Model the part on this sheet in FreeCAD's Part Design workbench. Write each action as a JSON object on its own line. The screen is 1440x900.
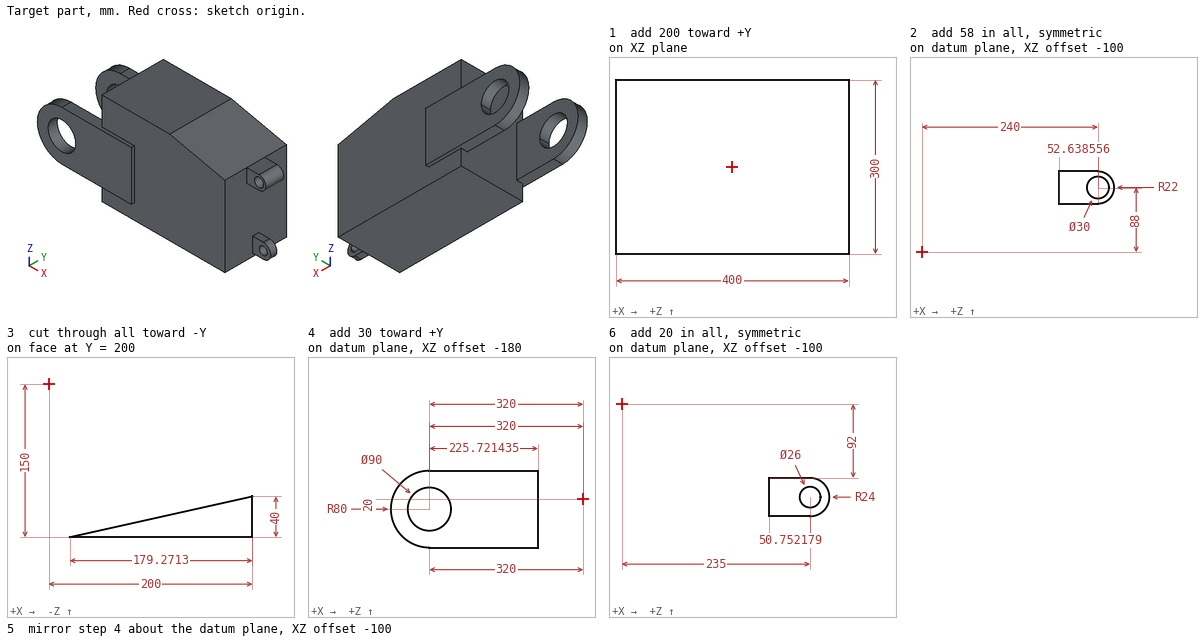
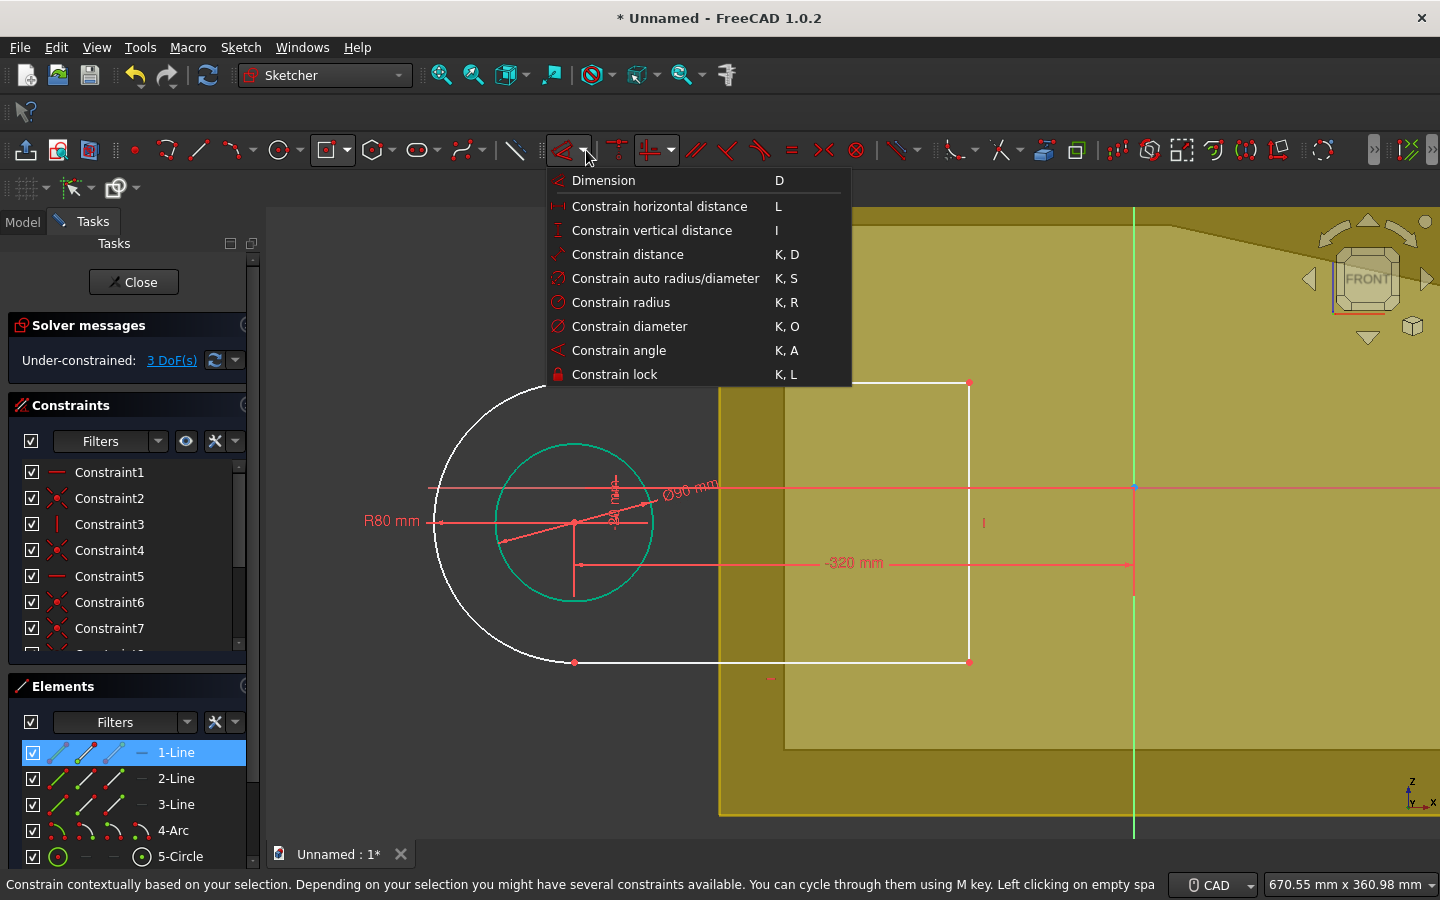
{"action": "left_click", "coordinate": [699, 206]}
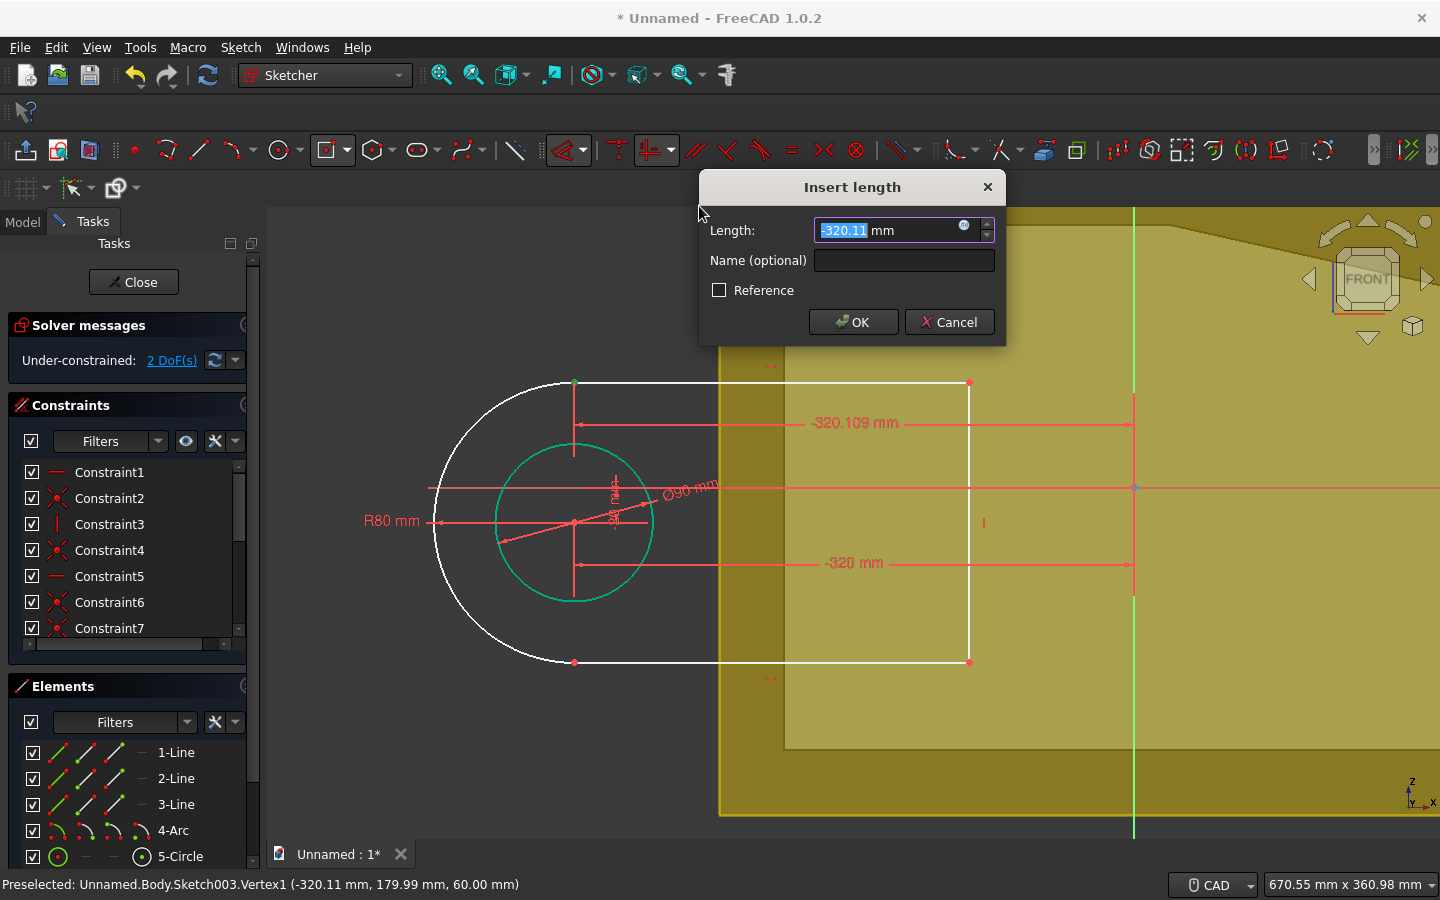
{"action": "type", "text": "-320"}
{"action": "key", "text": "Return"}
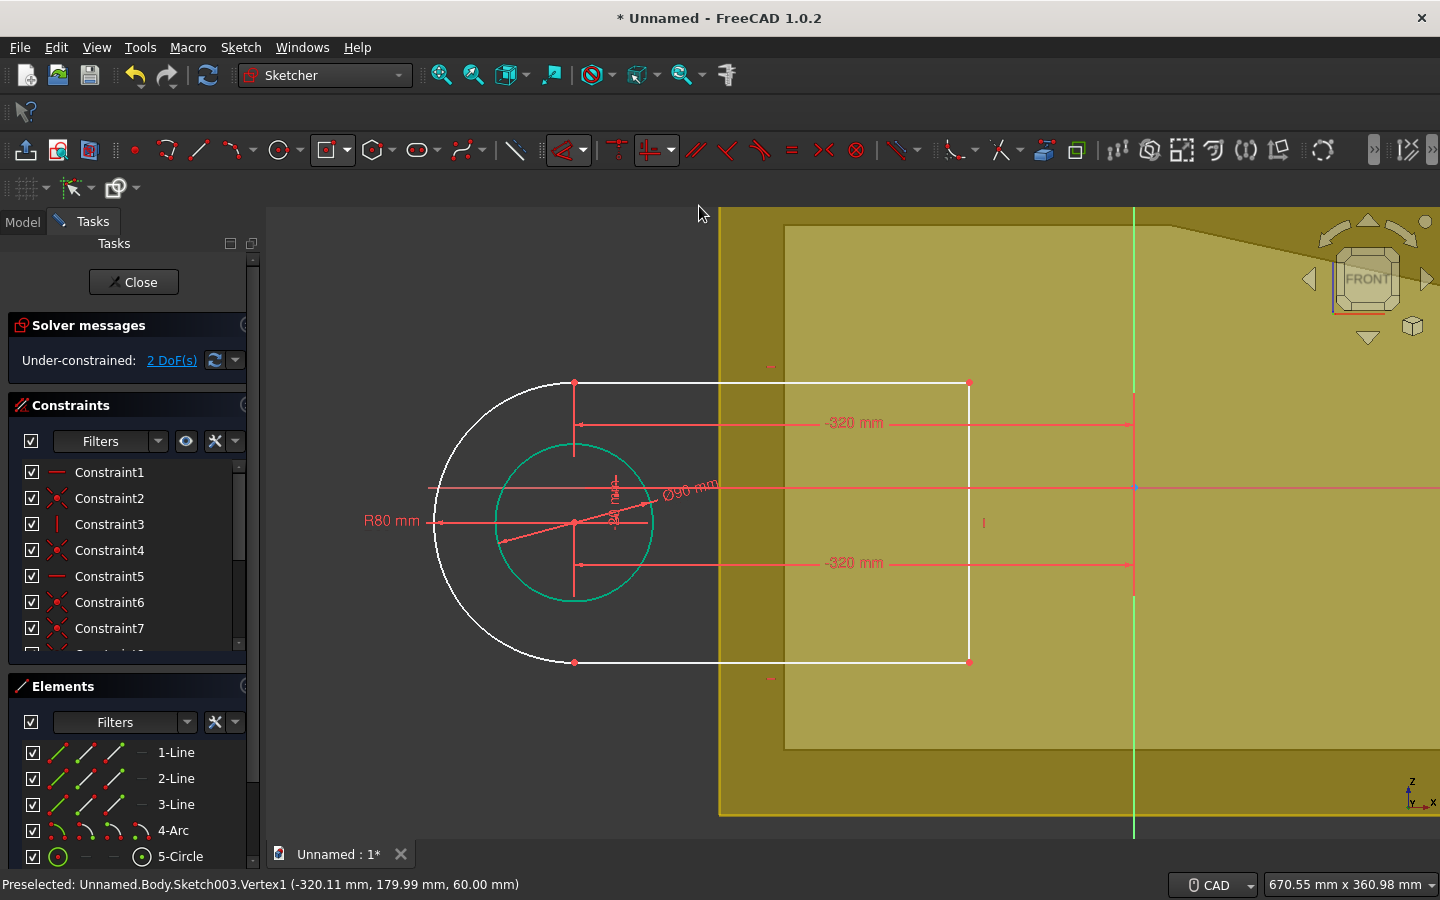
{"action": "left_click", "coordinate": [574, 663]}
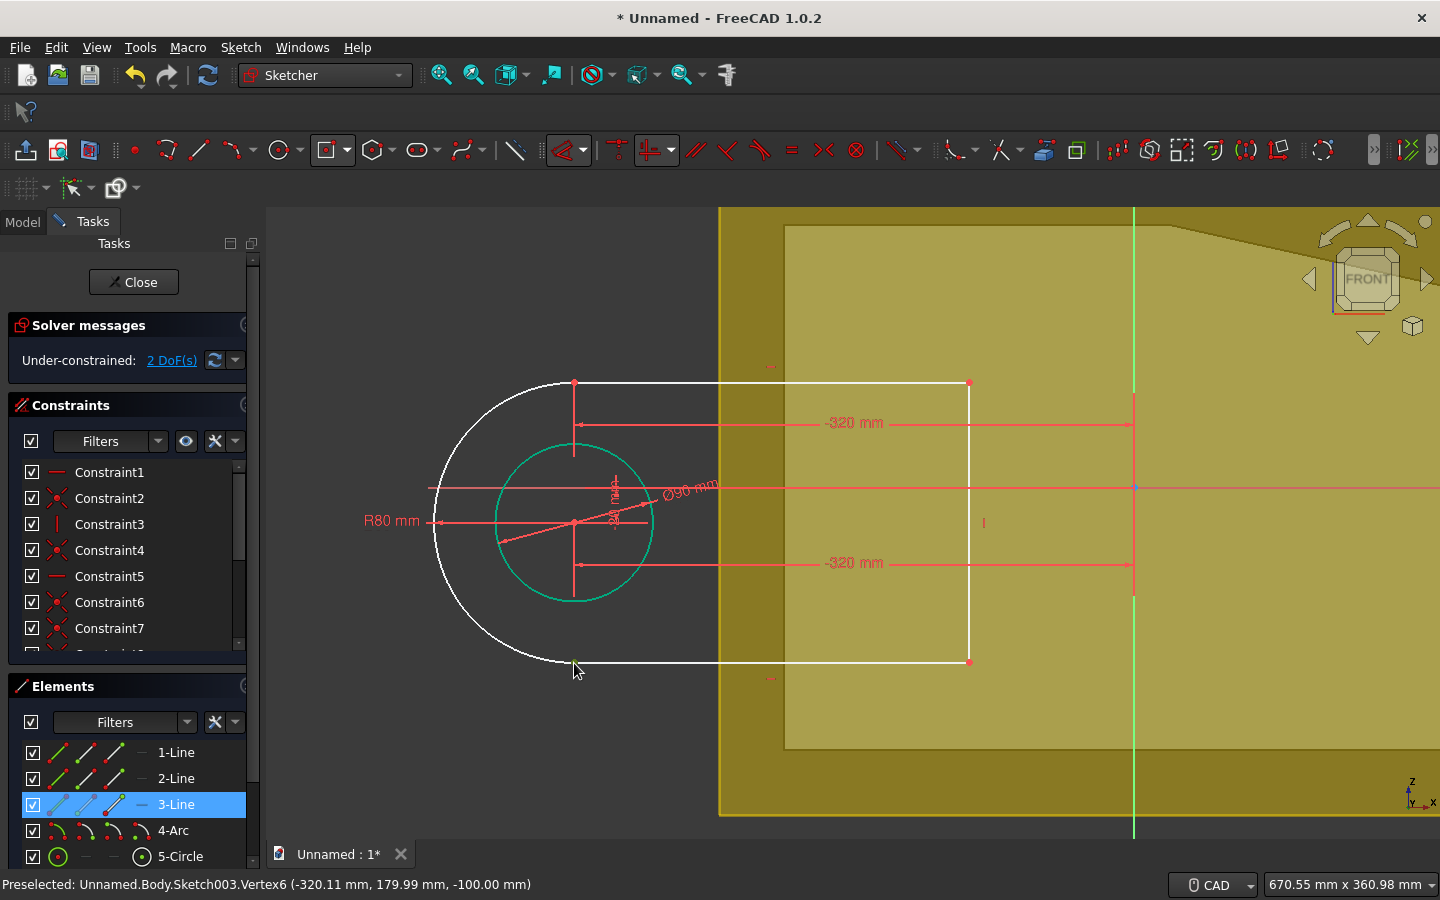
{"action": "left_click", "coordinate": [586, 150]}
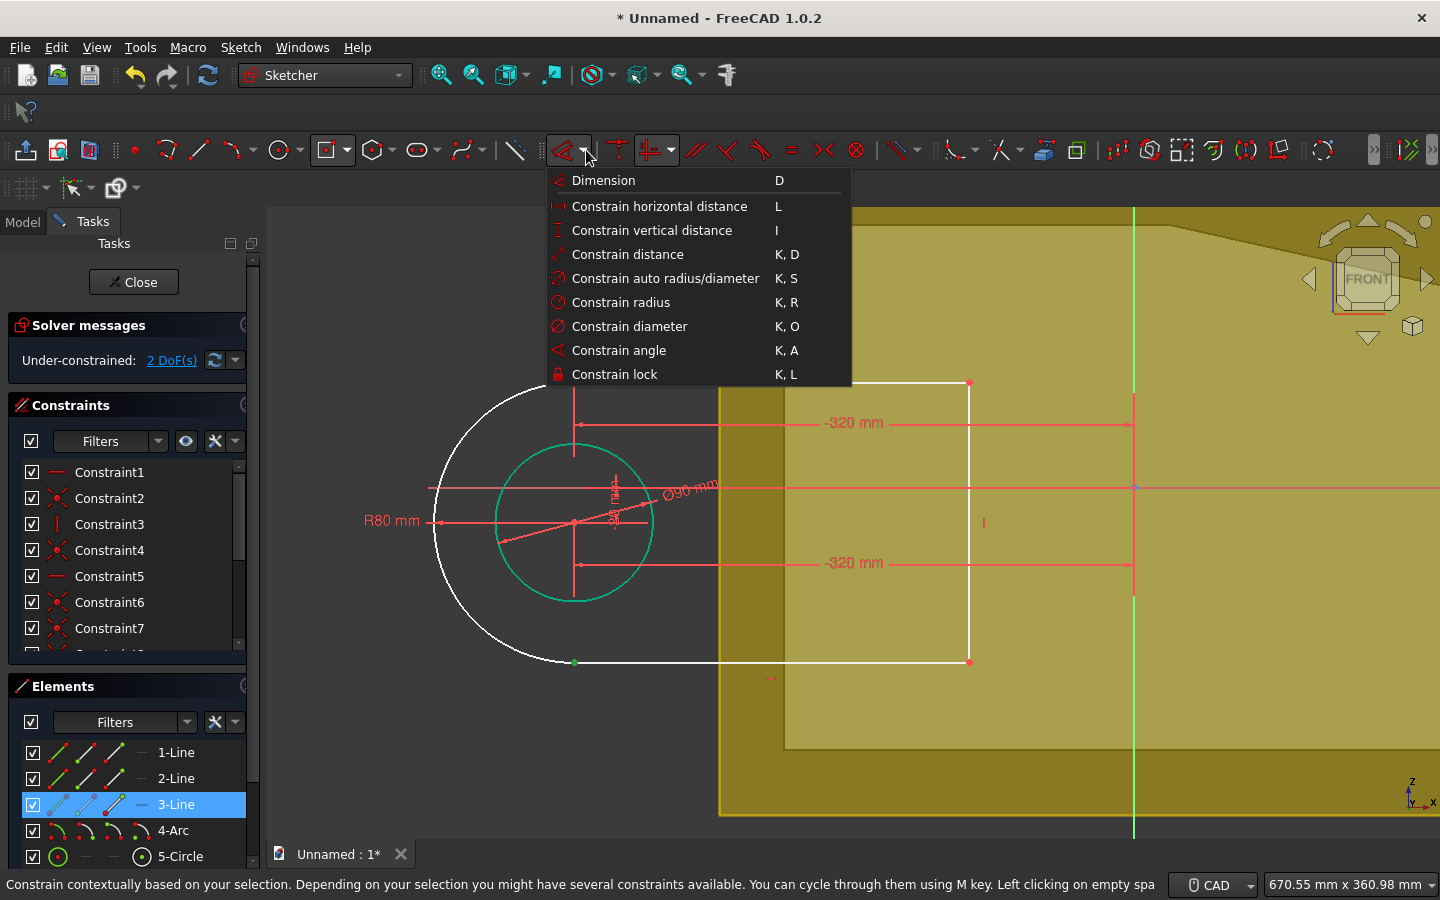
{"action": "left_click", "coordinate": [699, 206]}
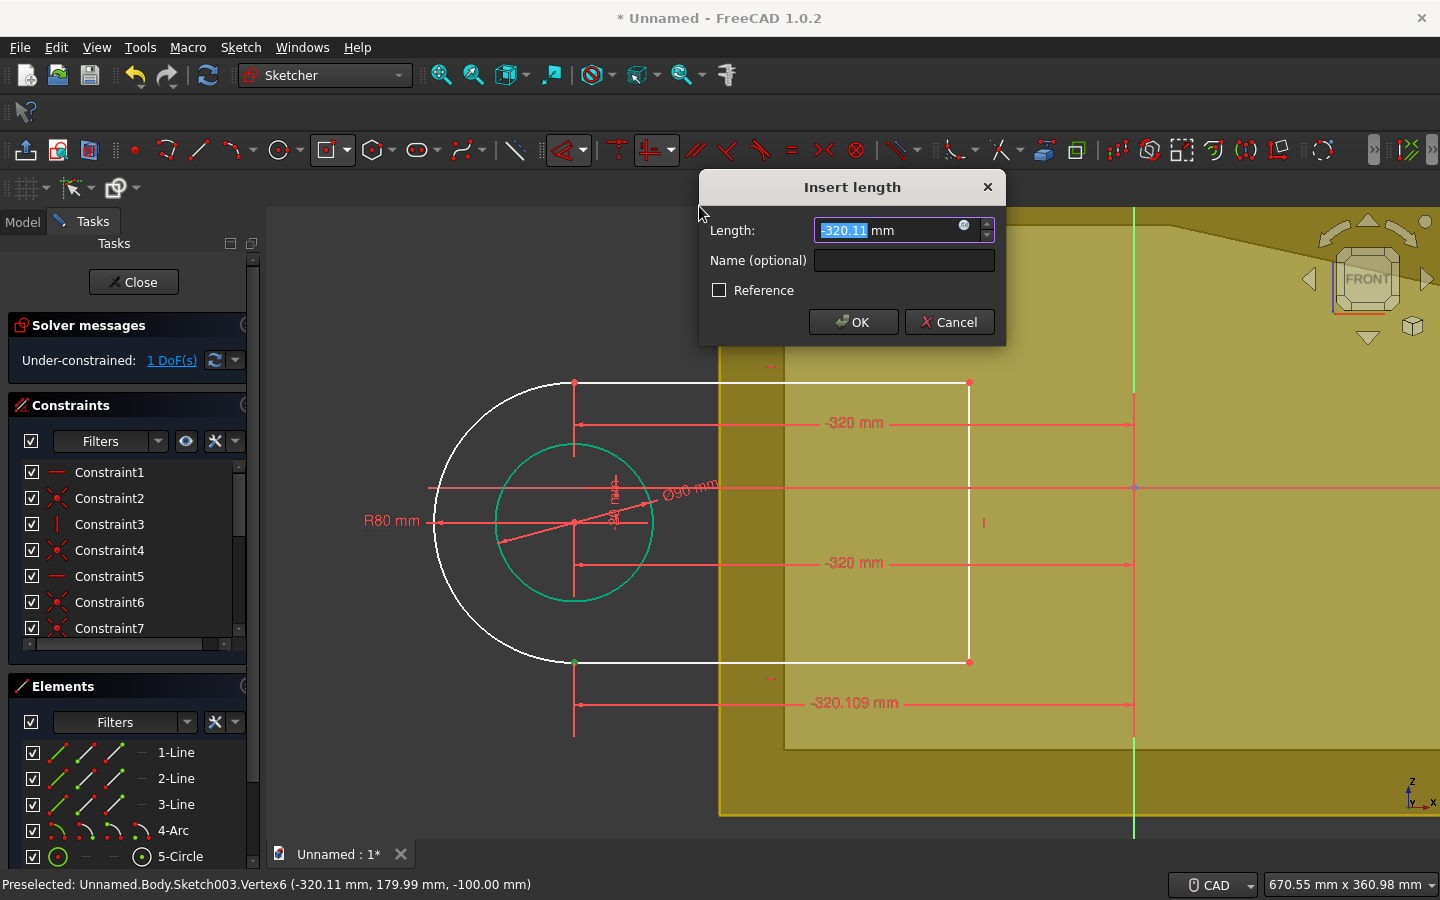
{"action": "type", "text": "-320"}
{"action": "key", "text": "Return"}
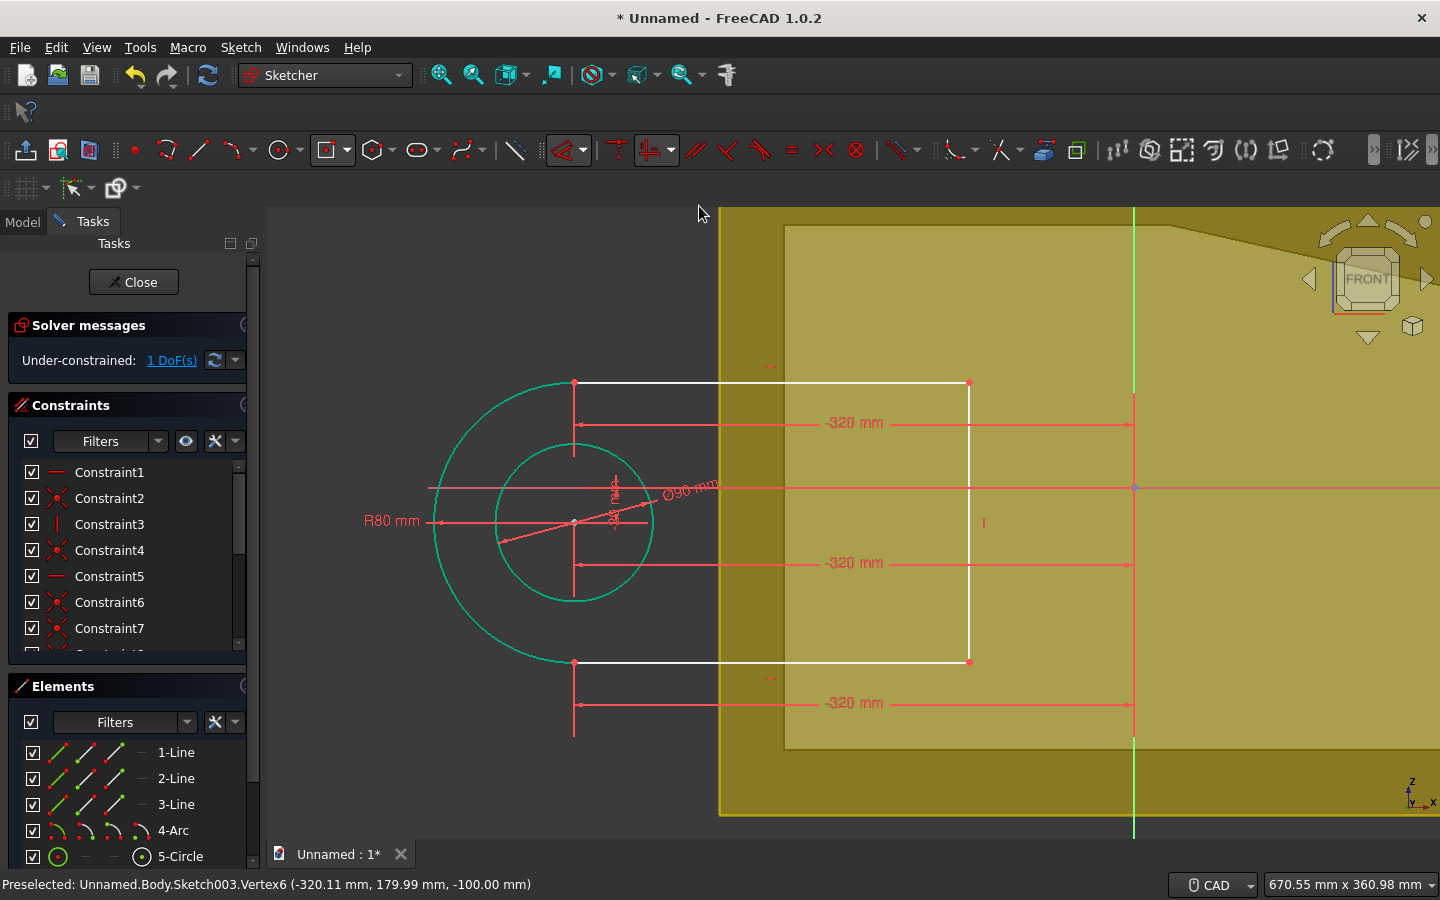
{"action": "left_click", "coordinate": [693, 383]}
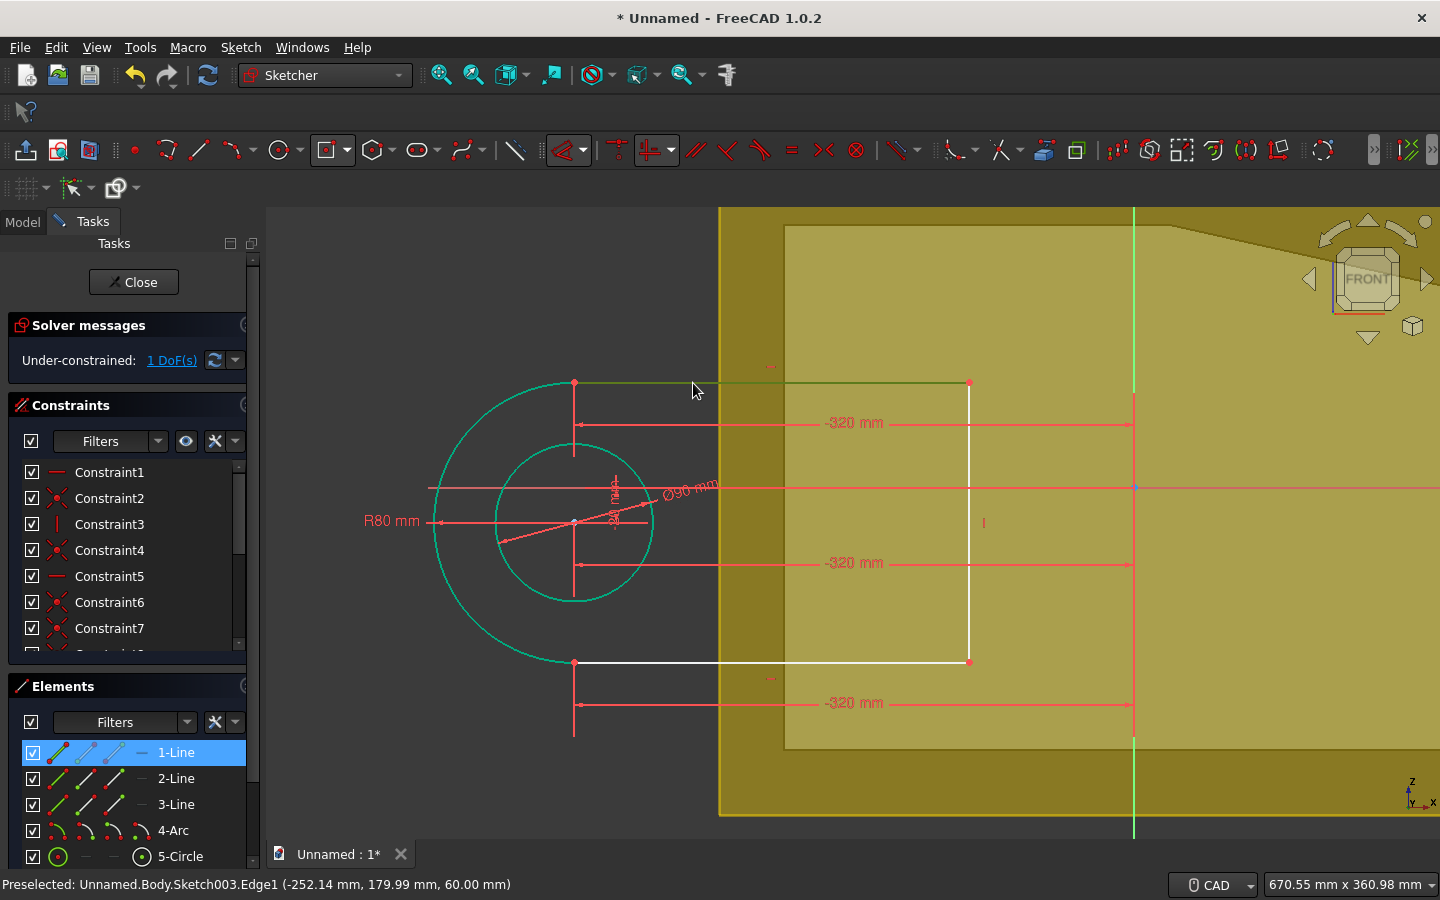
{"action": "left_click", "coordinate": [586, 150]}